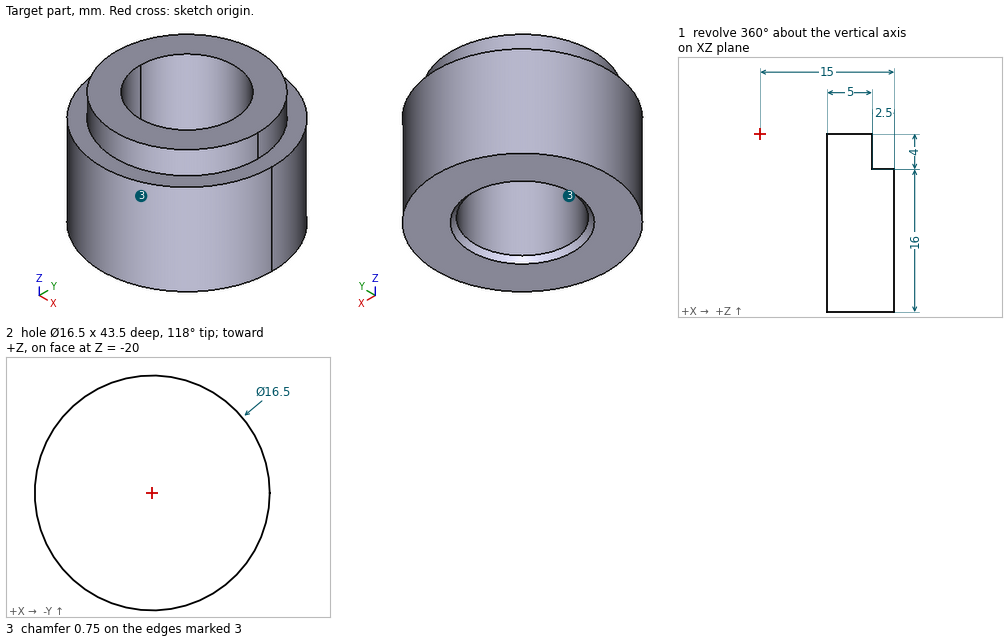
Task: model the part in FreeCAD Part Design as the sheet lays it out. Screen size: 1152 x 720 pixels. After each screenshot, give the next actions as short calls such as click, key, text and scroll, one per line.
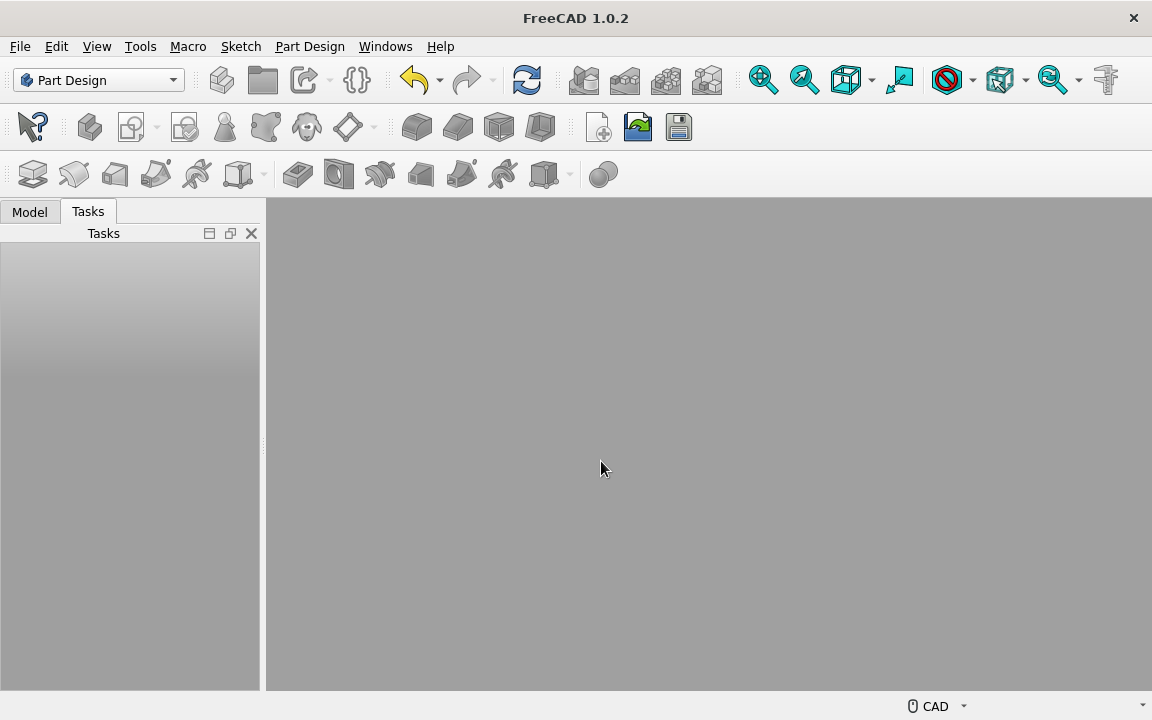
click(597, 128)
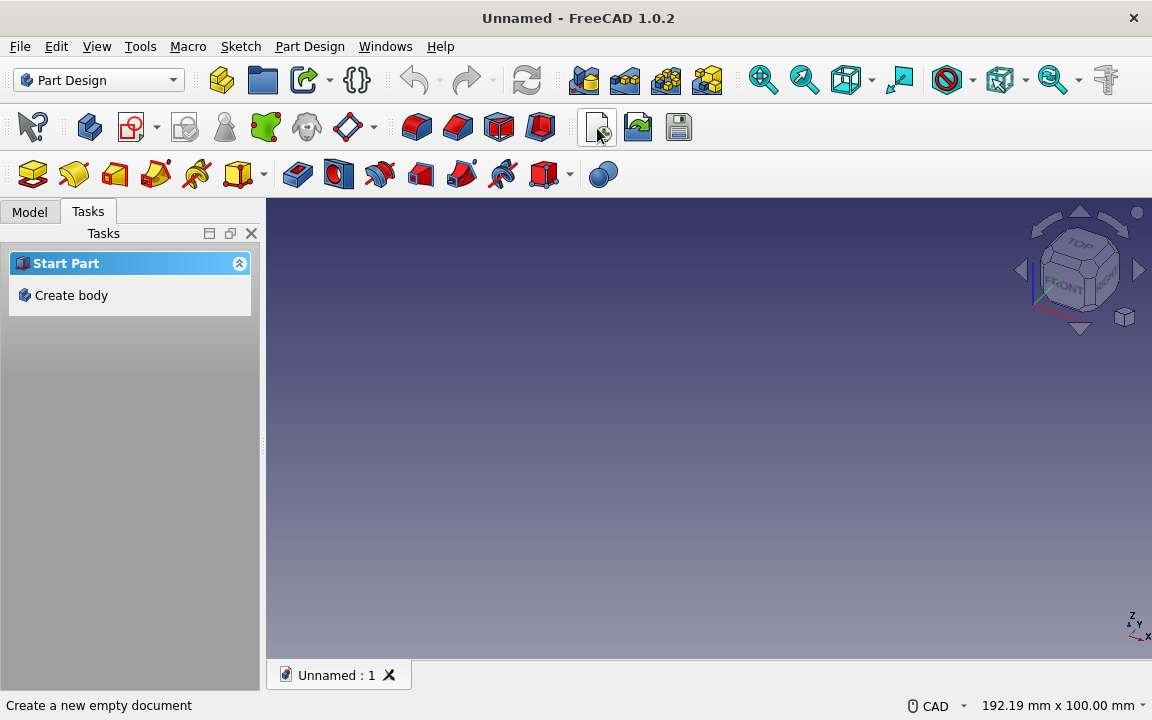
click(130, 128)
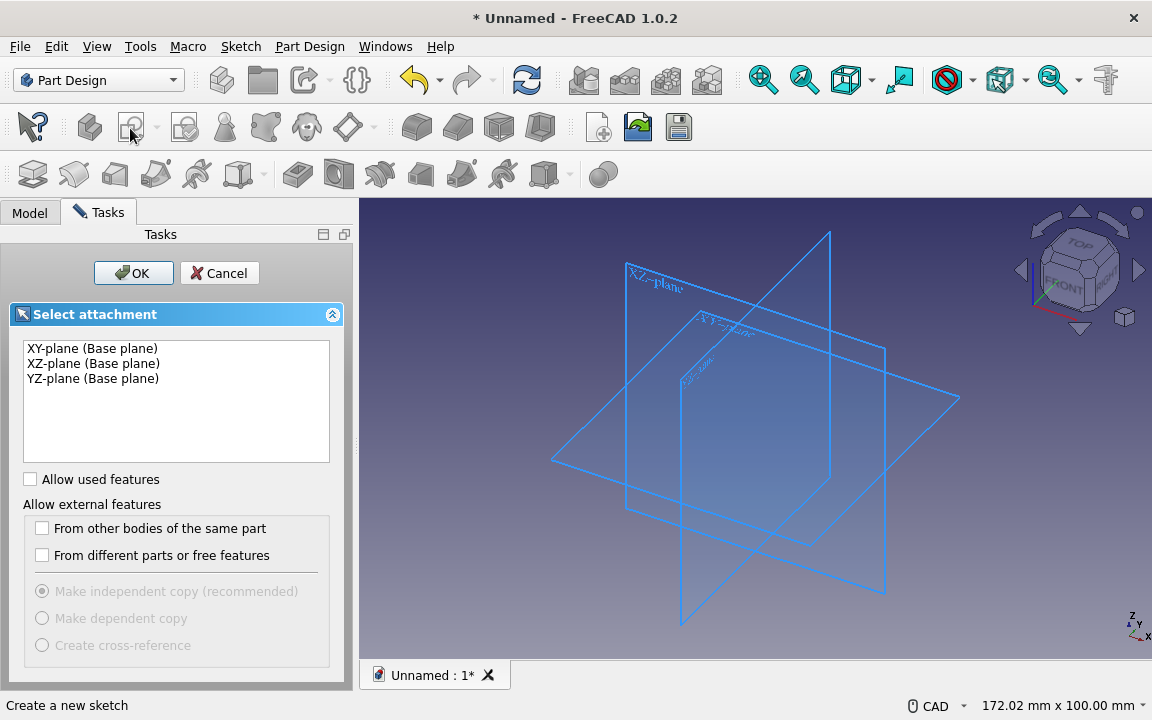
click(84, 364)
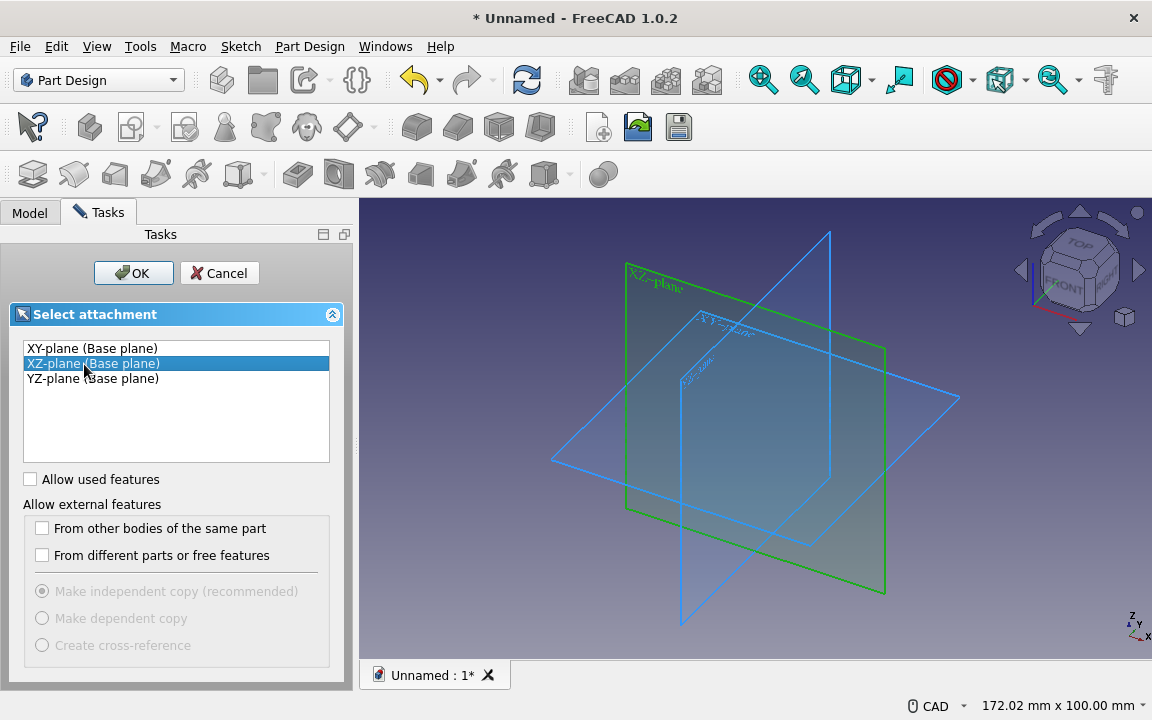
click(134, 273)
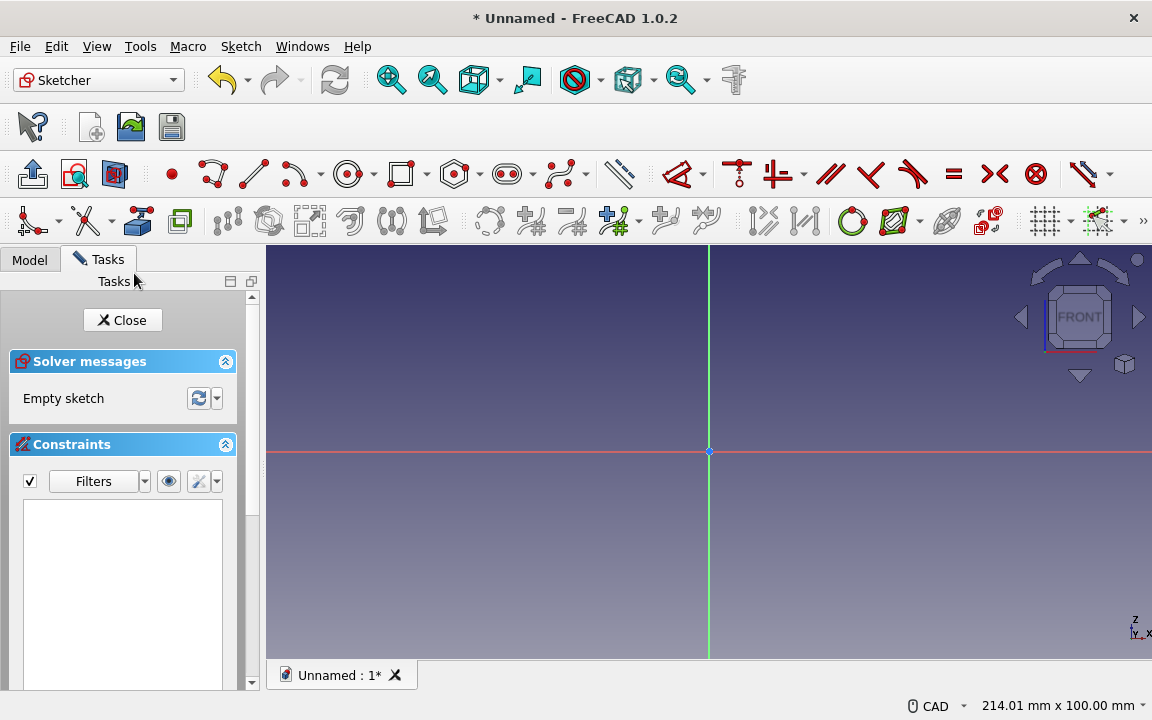
scroll(783, 511, up, 6)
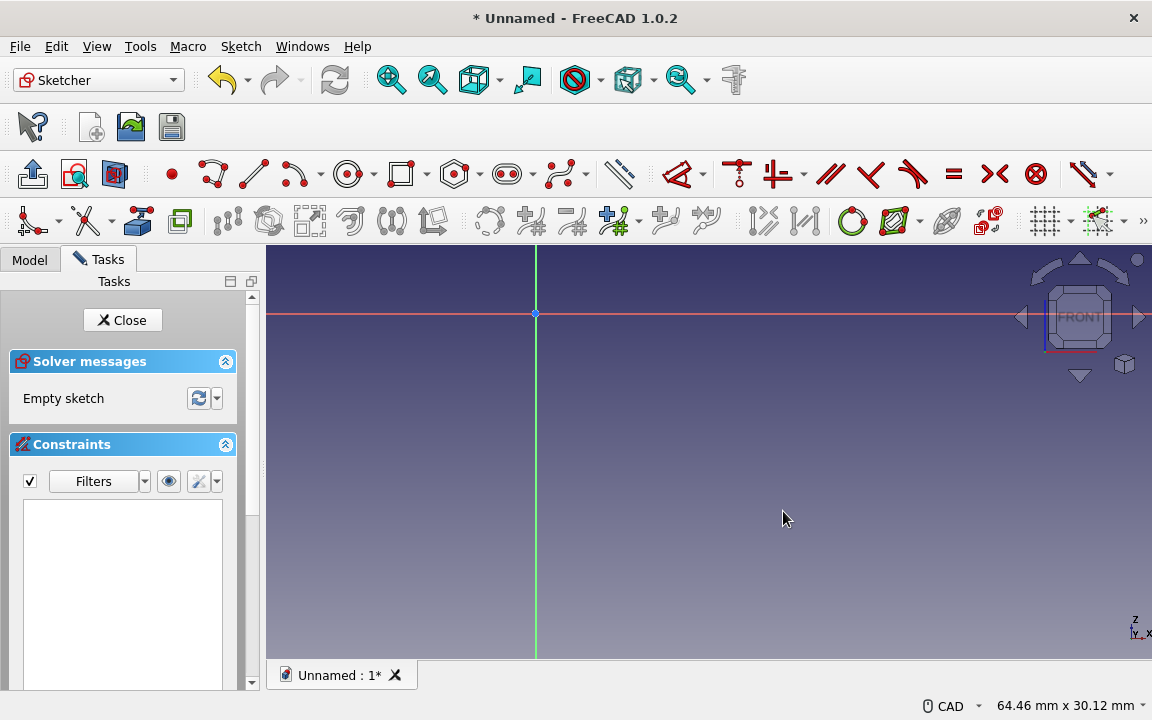
click(213, 174)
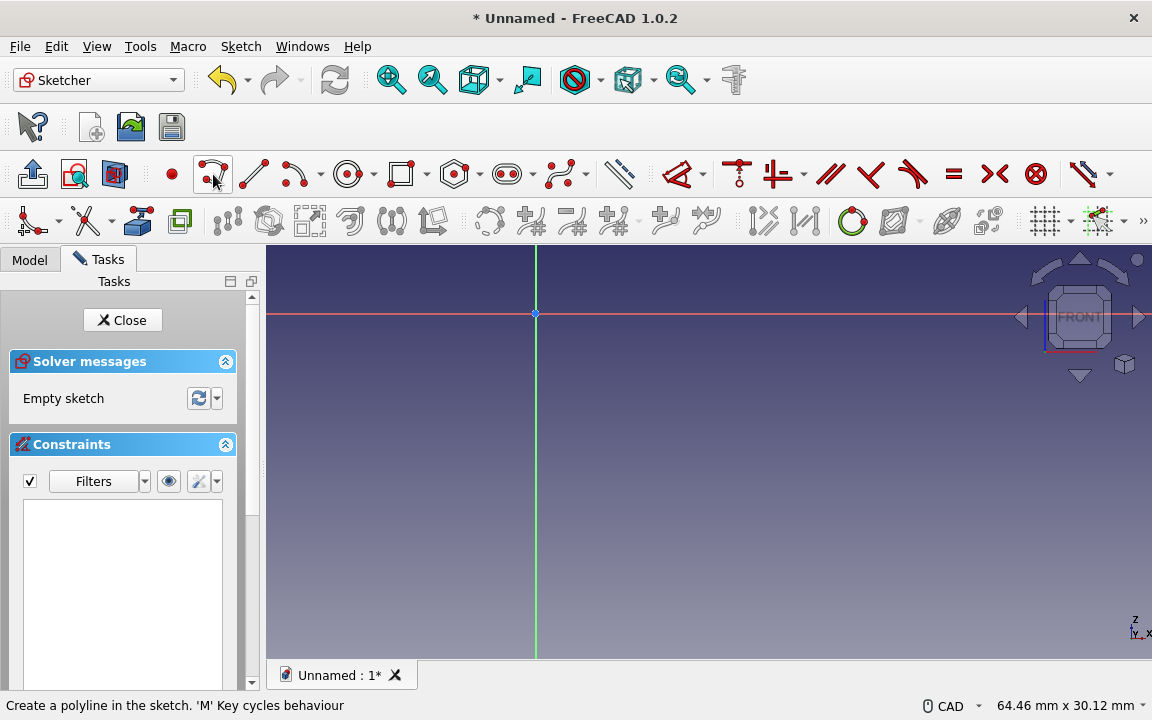
click(639, 314)
click(708, 323)
click(708, 369)
click(742, 369)
click(742, 589)
click(639, 589)
click(639, 314)
key(Escape)
key(Escape)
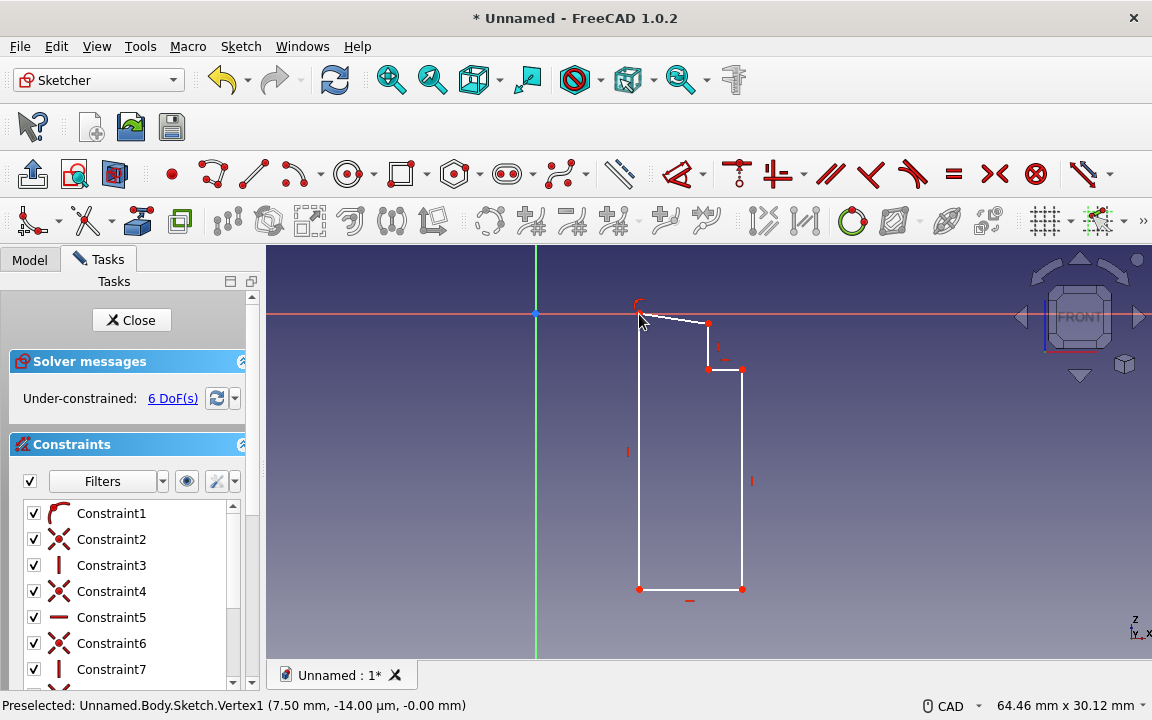
click(660, 317)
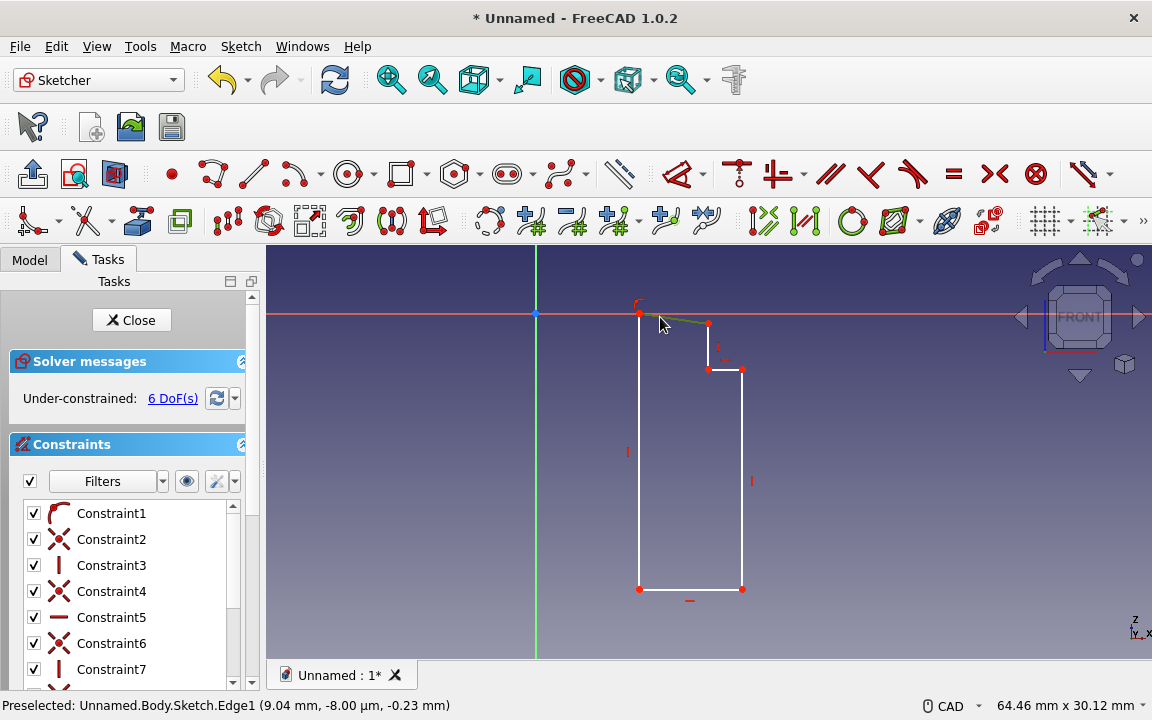
click(804, 174)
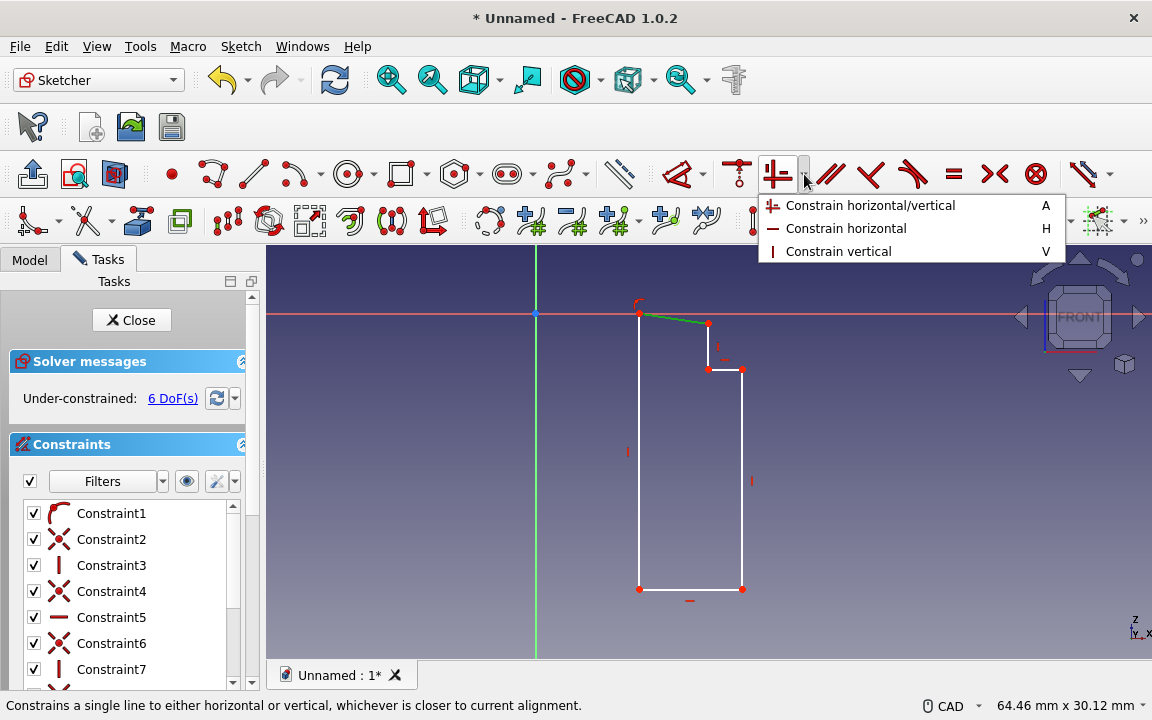
click(912, 228)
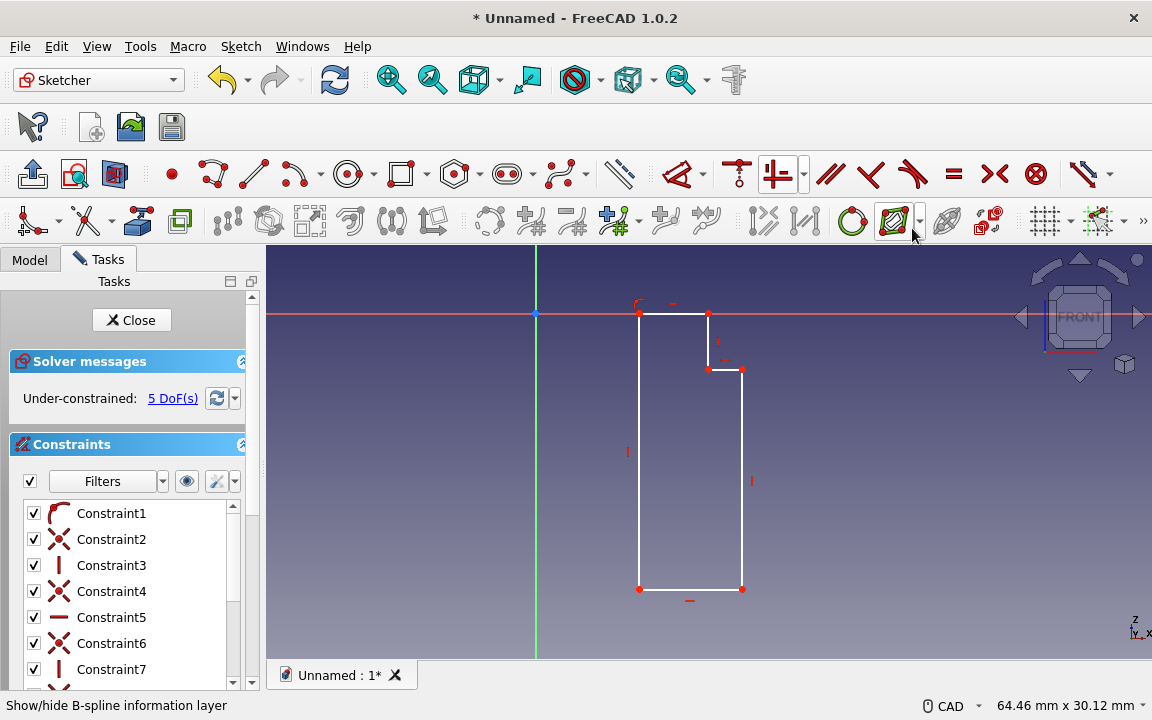
click(676, 174)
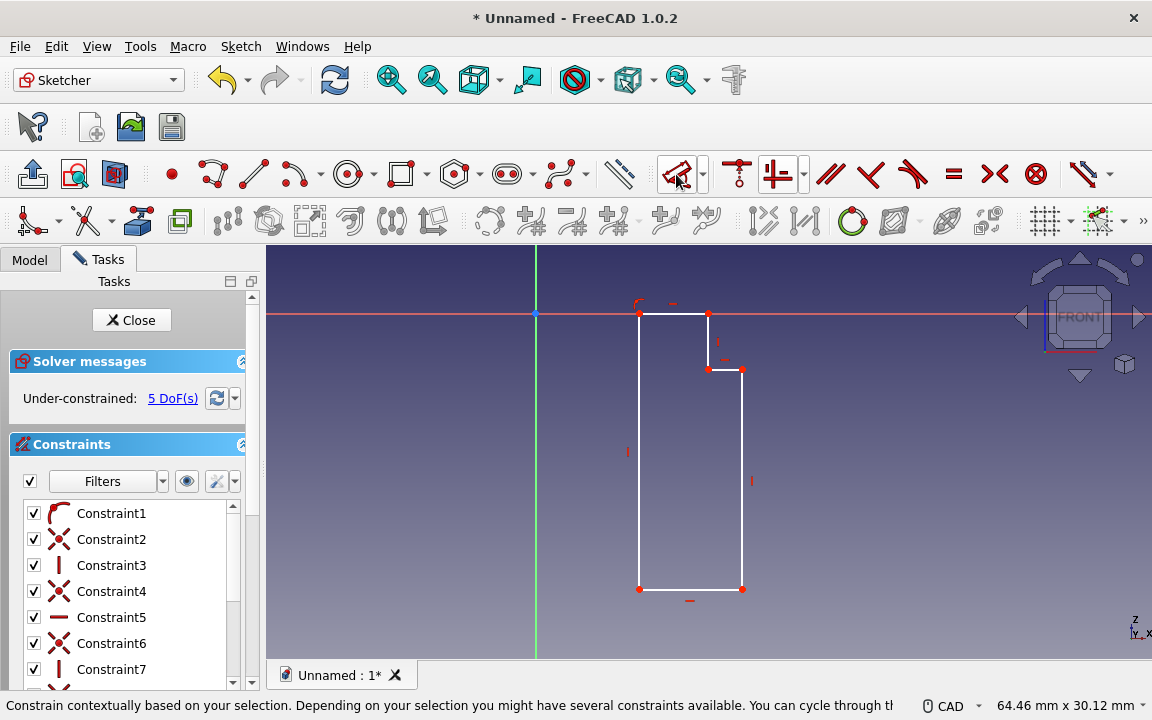
click(660, 314)
click(674, 280)